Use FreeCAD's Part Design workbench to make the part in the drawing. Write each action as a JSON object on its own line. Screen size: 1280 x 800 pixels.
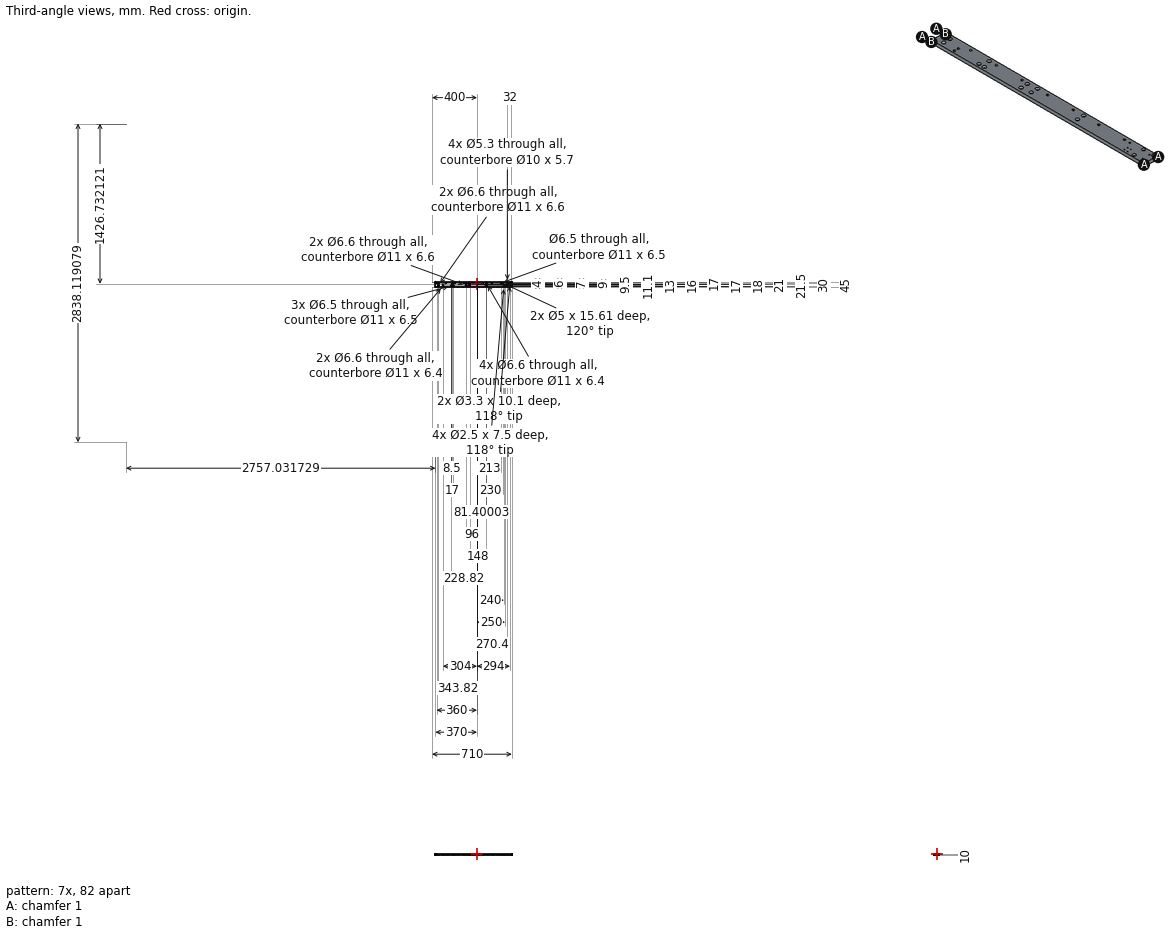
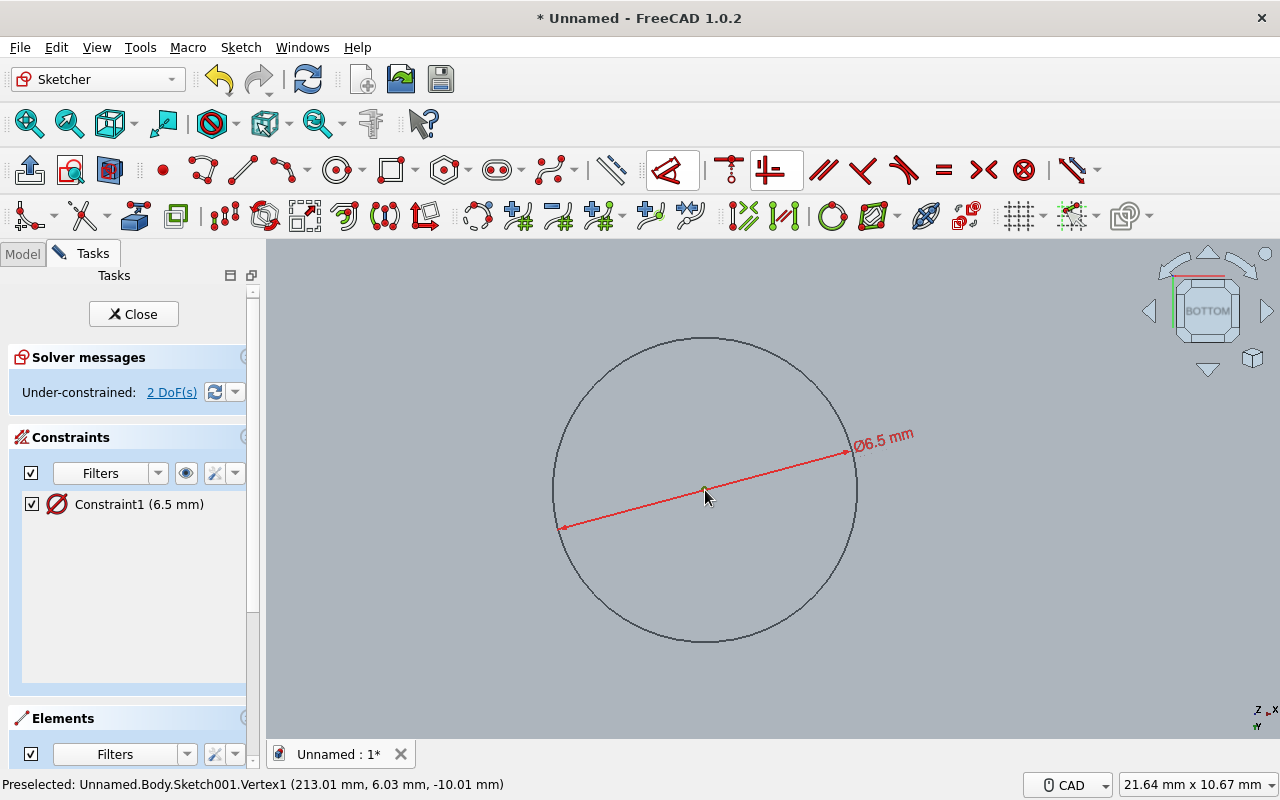
{"action": "left_click", "coordinate": [694, 170]}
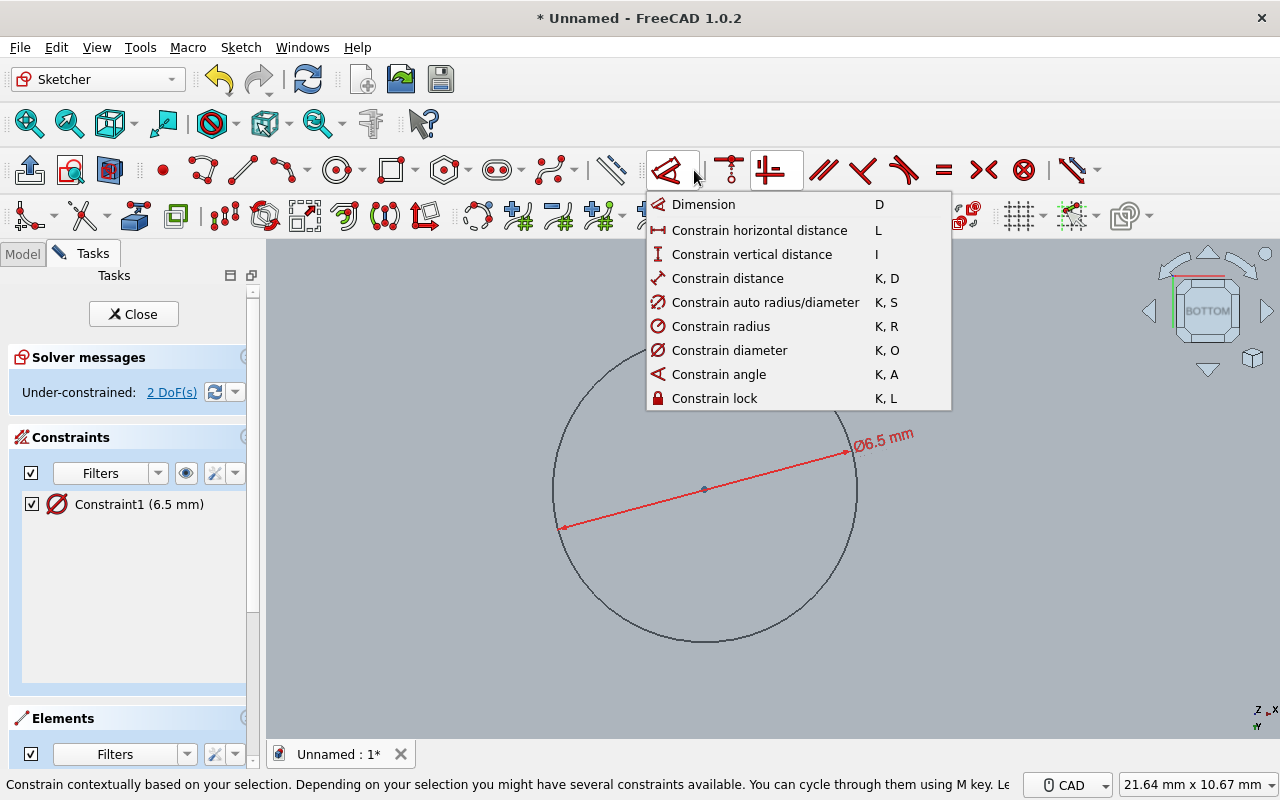
{"action": "left_click", "coordinate": [799, 254]}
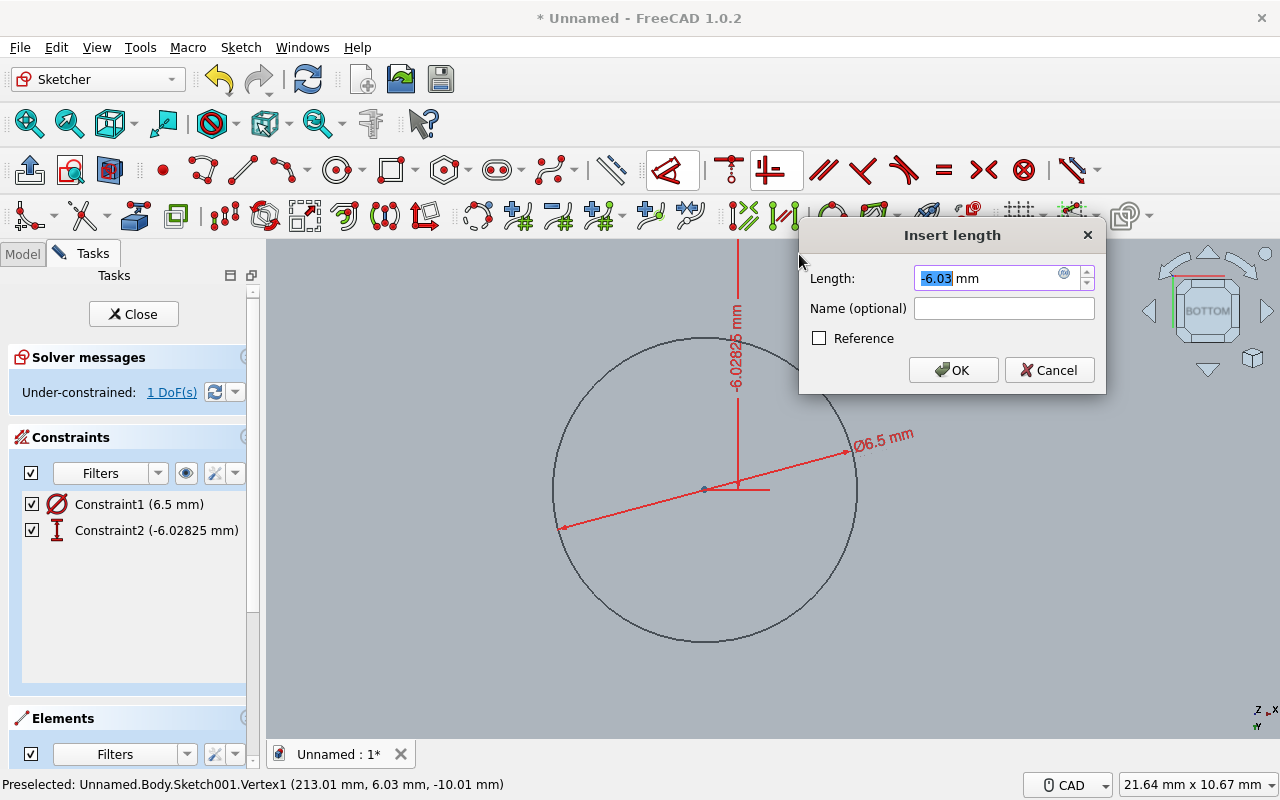
{"action": "type", "text": "-6"}
{"action": "key", "text": "Return"}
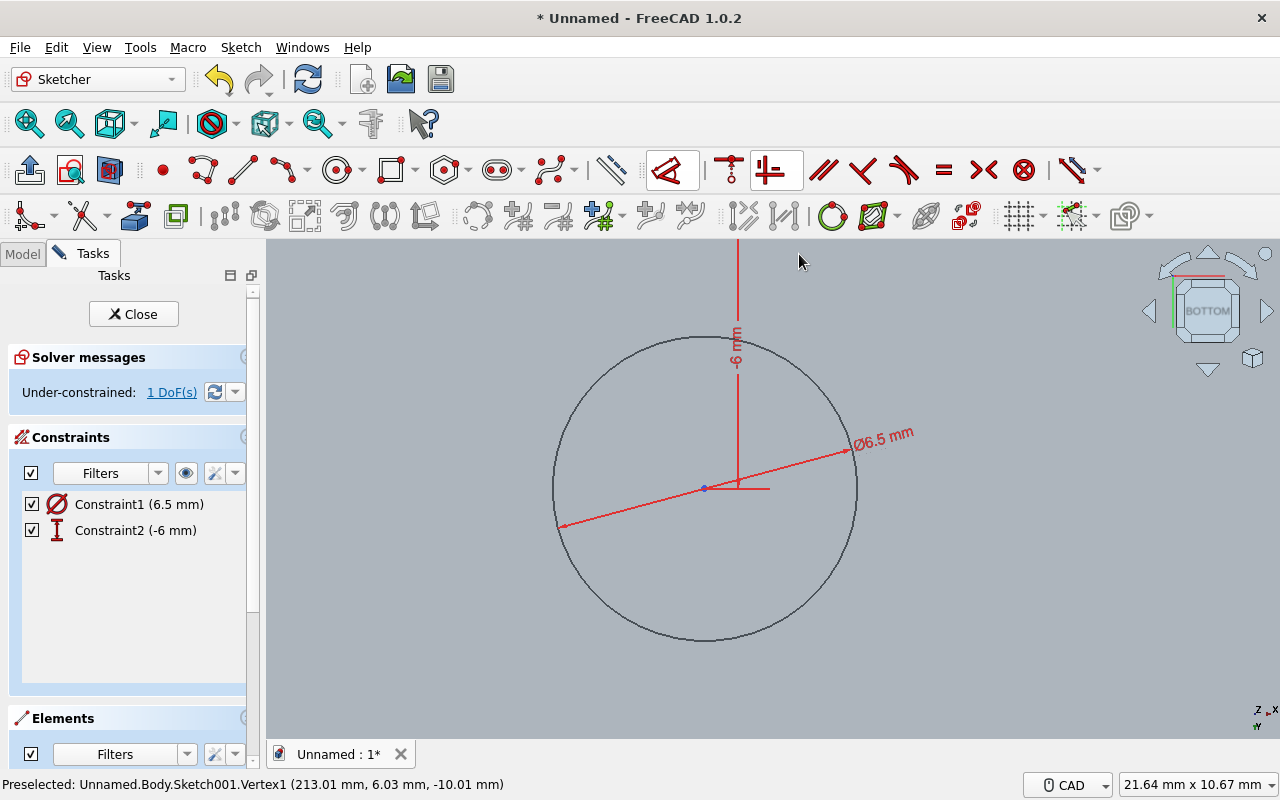
{"action": "left_click", "coordinate": [705, 489]}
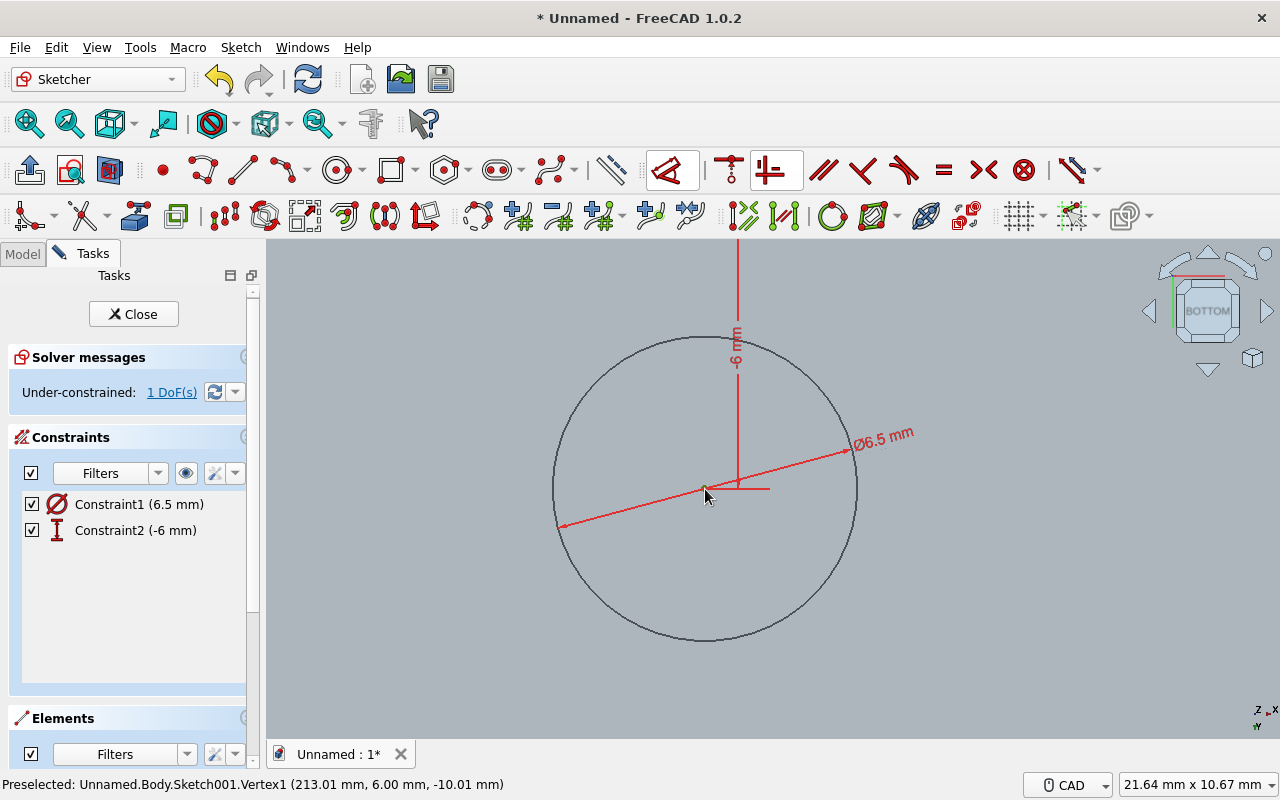
{"action": "key", "text": "l"}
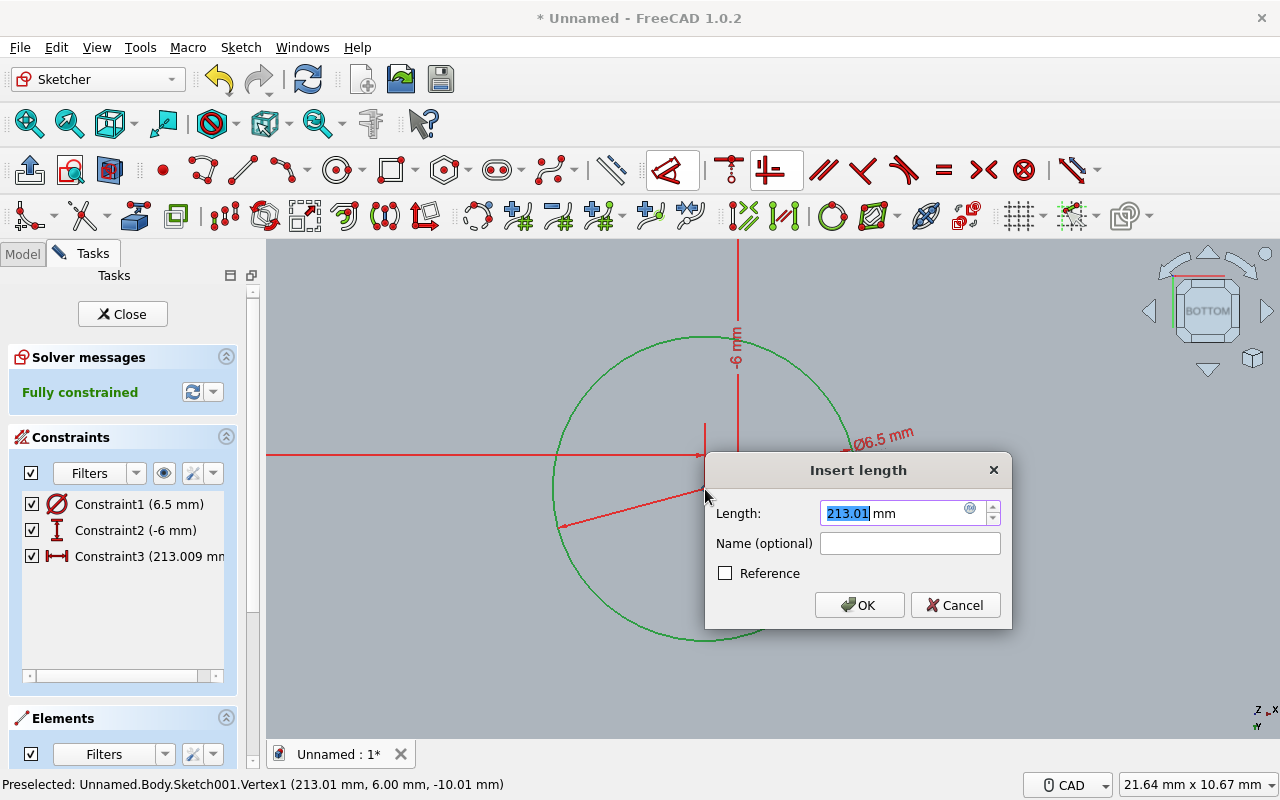
{"action": "type", "text": "213"}
{"action": "key", "text": "Return"}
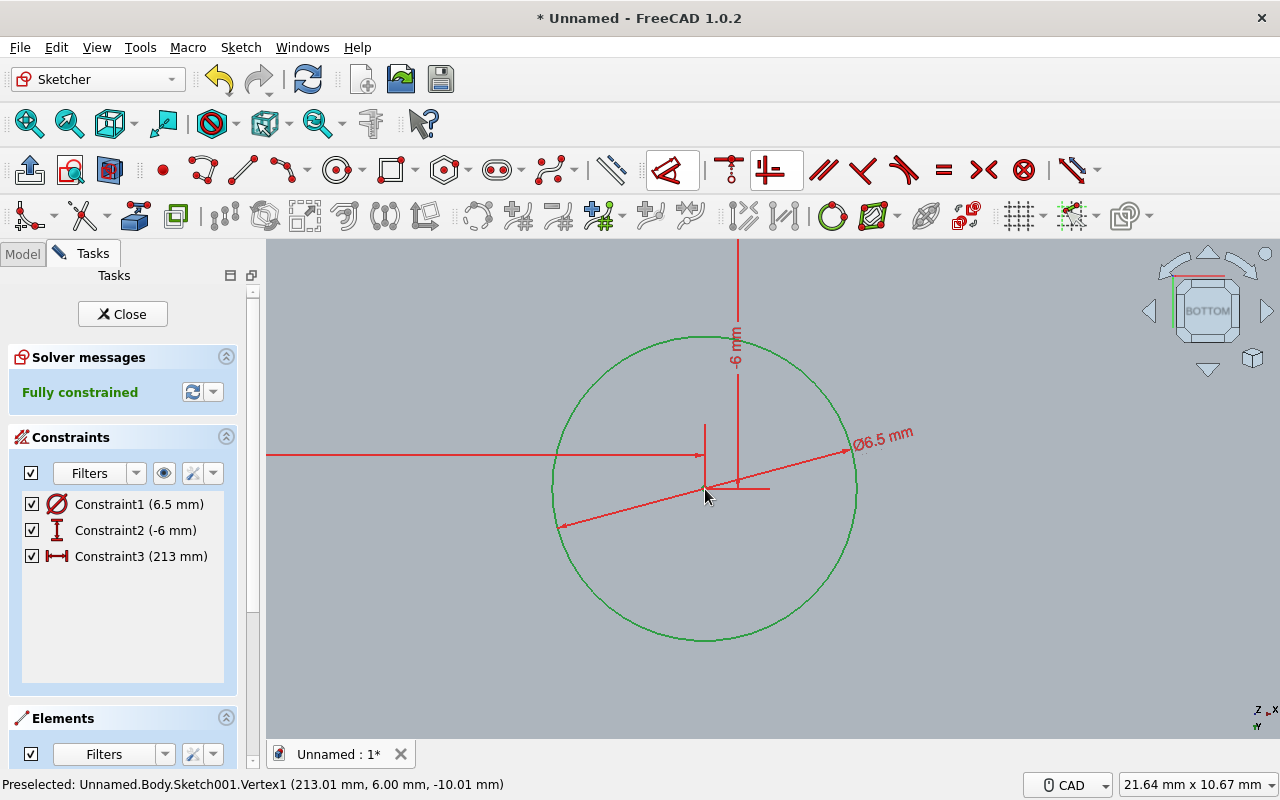
{"action": "left_click", "coordinate": [123, 314]}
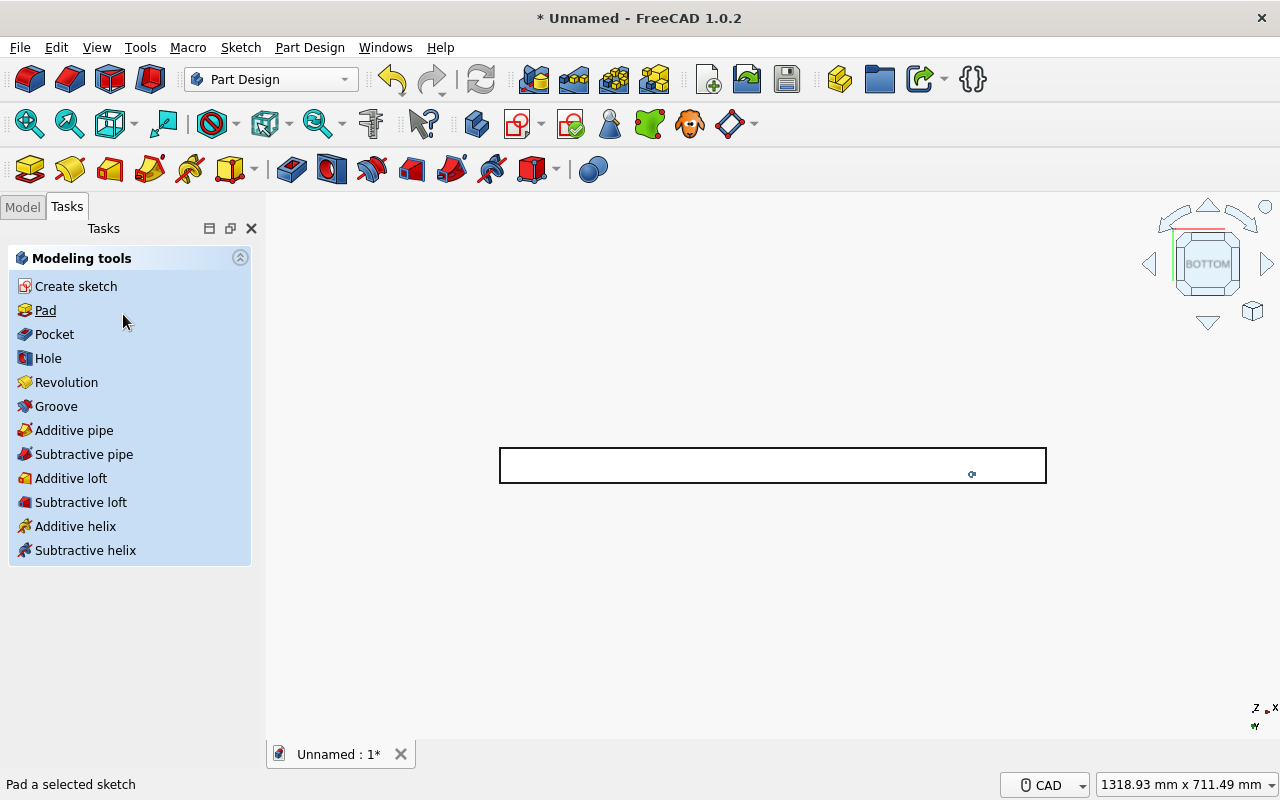
{"action": "left_click", "coordinate": [332, 170]}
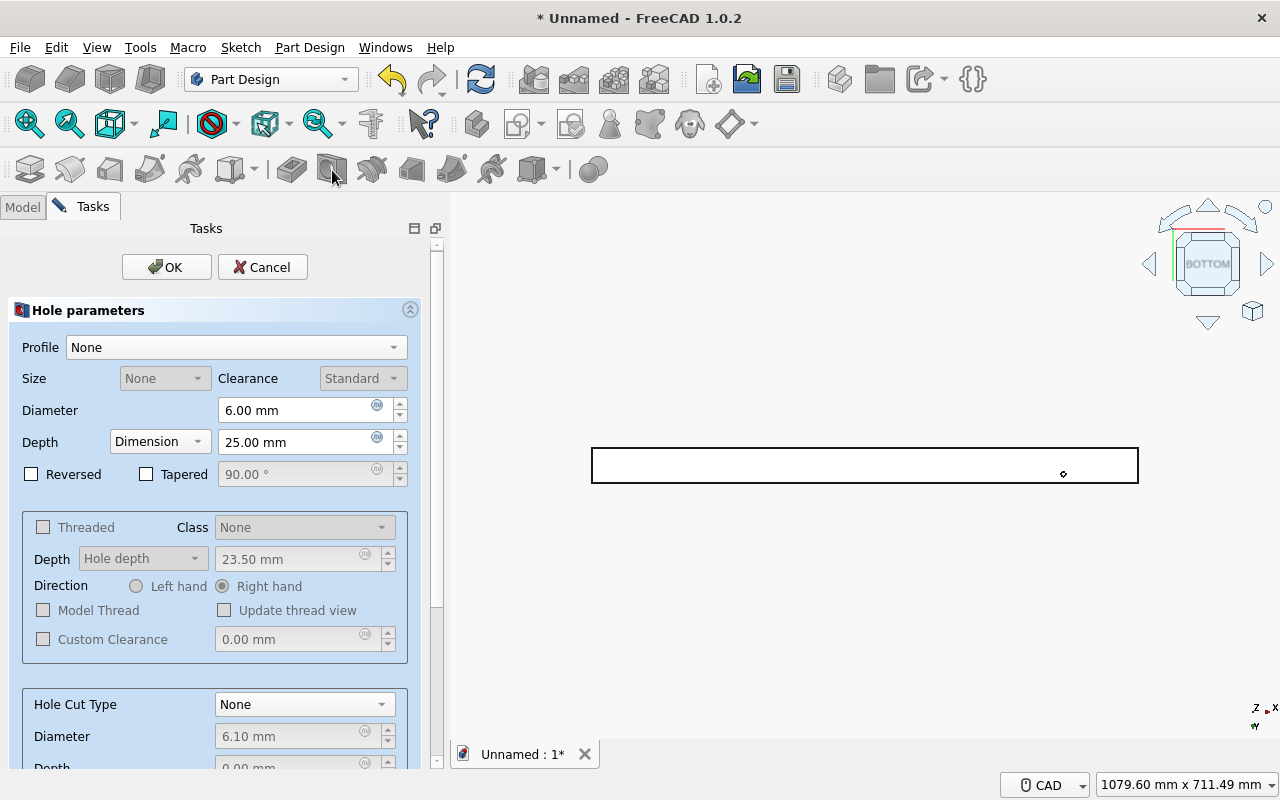
{"action": "triple_click", "coordinate": [305, 410]}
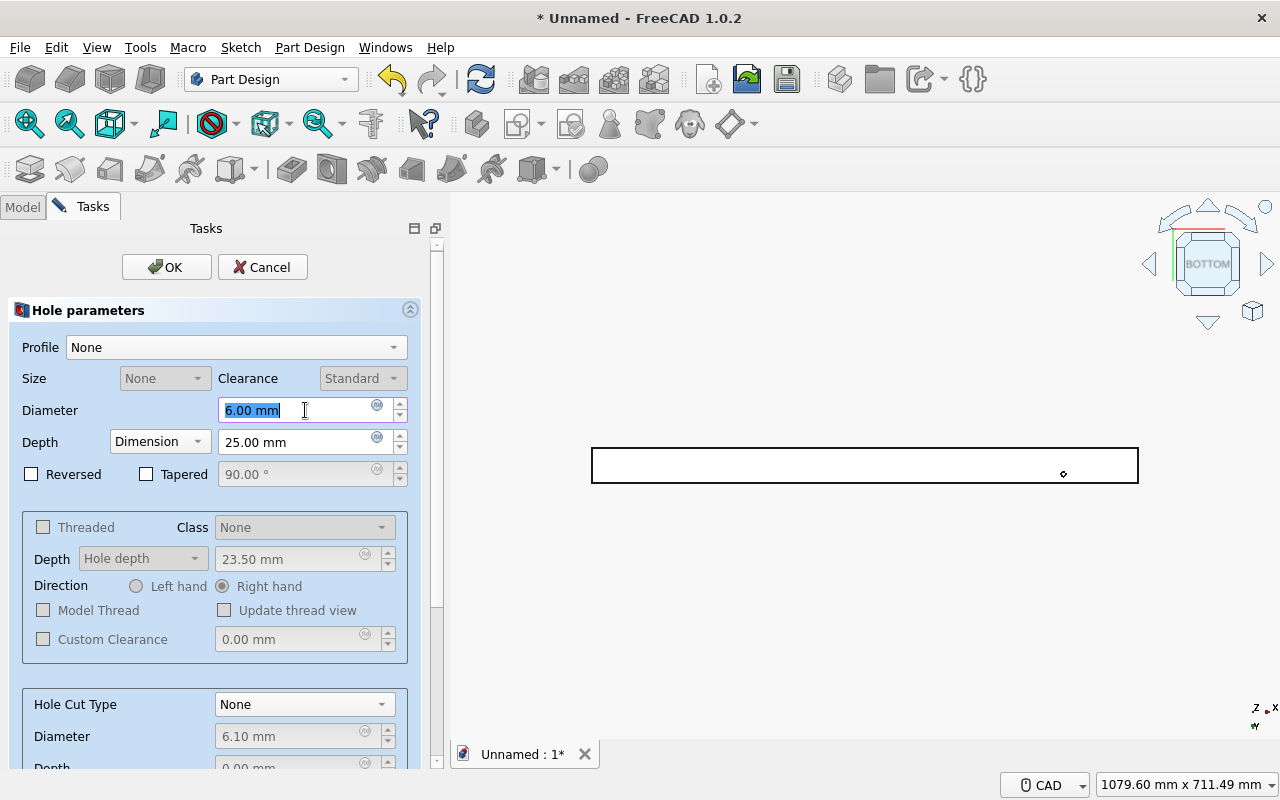
{"action": "type", "text": "6.5"}
{"action": "key", "text": "Tab"}